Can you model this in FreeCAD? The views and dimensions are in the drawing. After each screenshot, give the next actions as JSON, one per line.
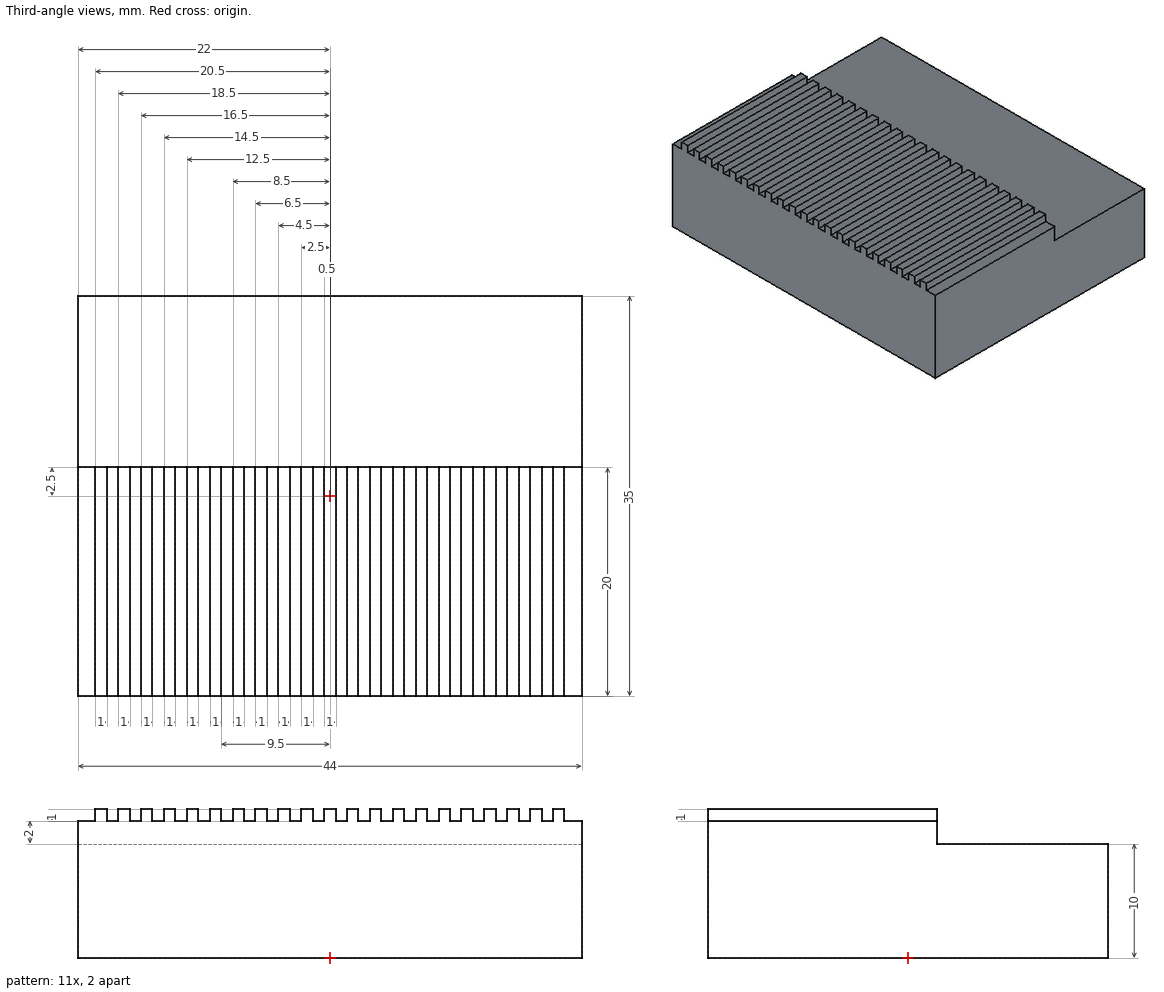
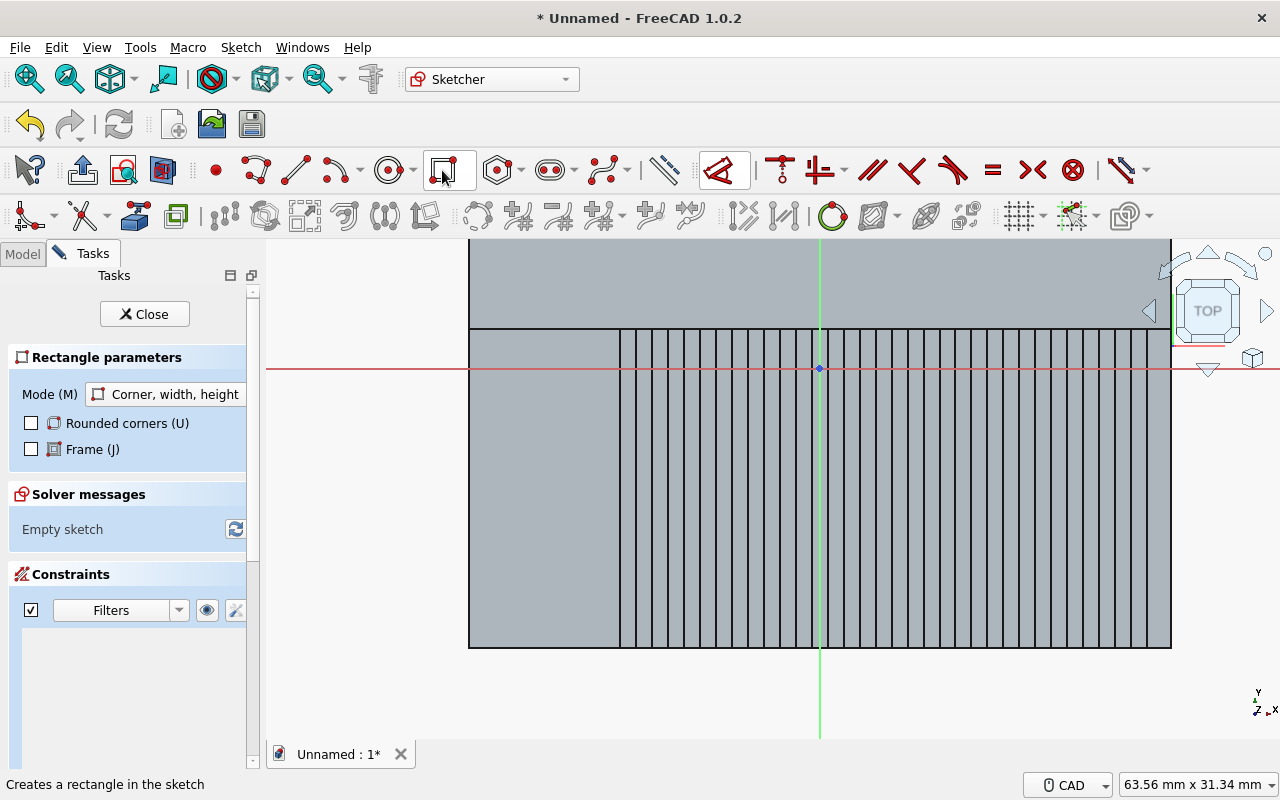
{"action": "left_click", "coordinate": [589, 329]}
{"action": "mouse_move", "coordinate": [604, 648]}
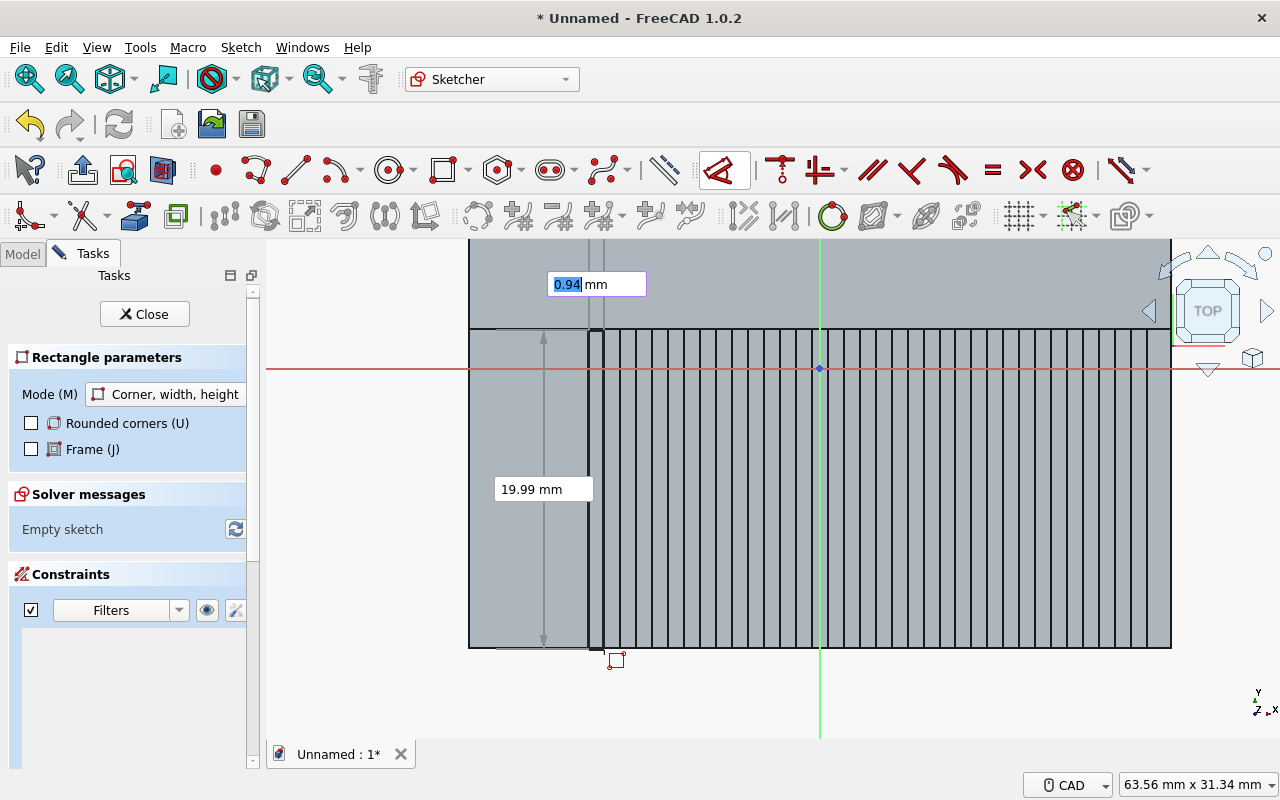
{"action": "type", "text": "1"}
{"action": "key", "text": "Tab"}
{"action": "type", "text": "20"}
{"action": "key", "text": "Return"}
{"action": "key", "text": "Escape"}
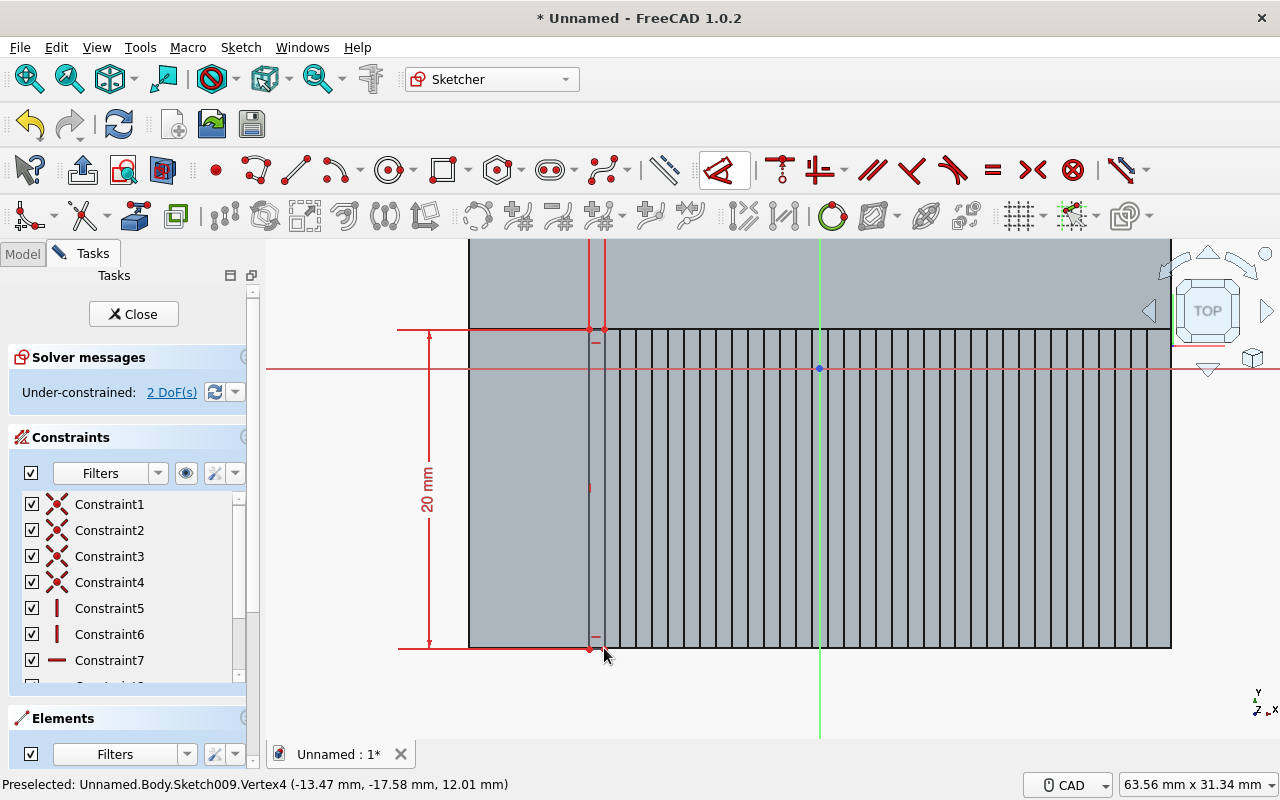
{"action": "left_click", "coordinate": [589, 330]}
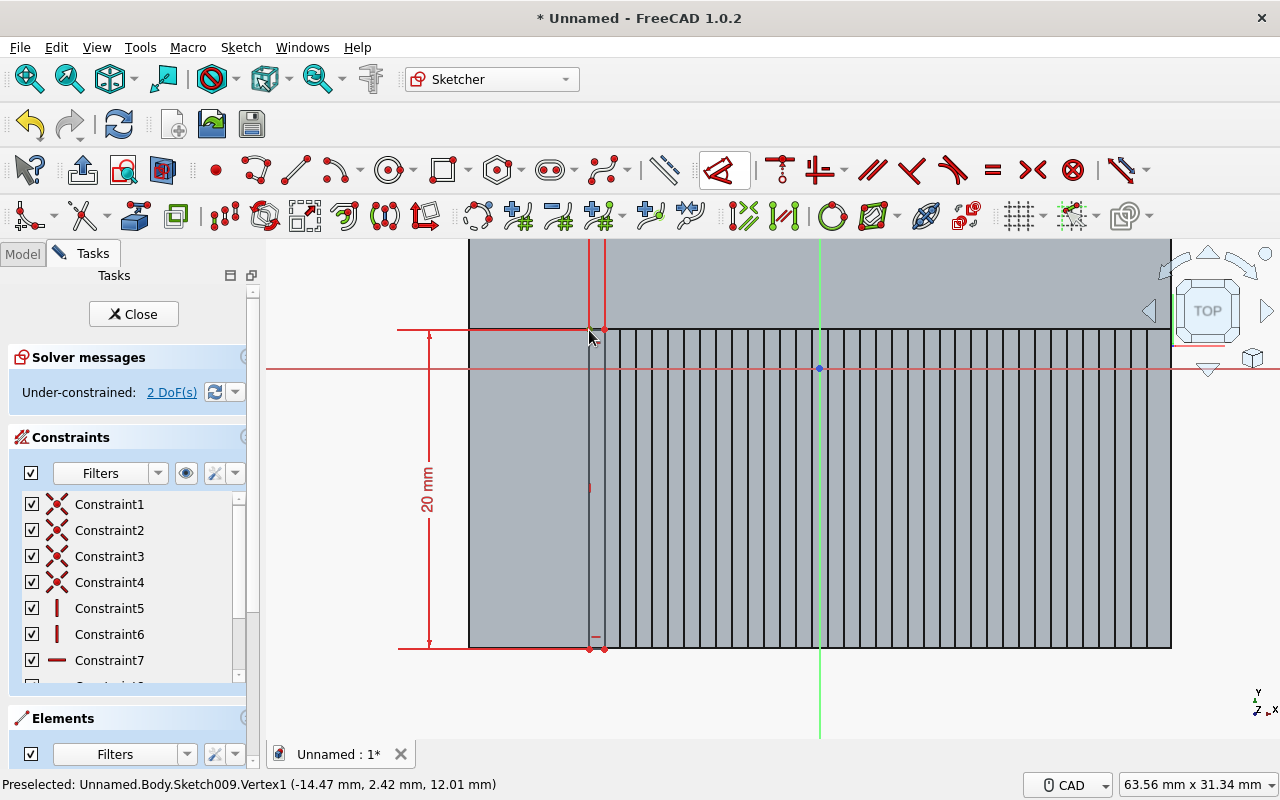
{"action": "left_click", "coordinate": [744, 170]}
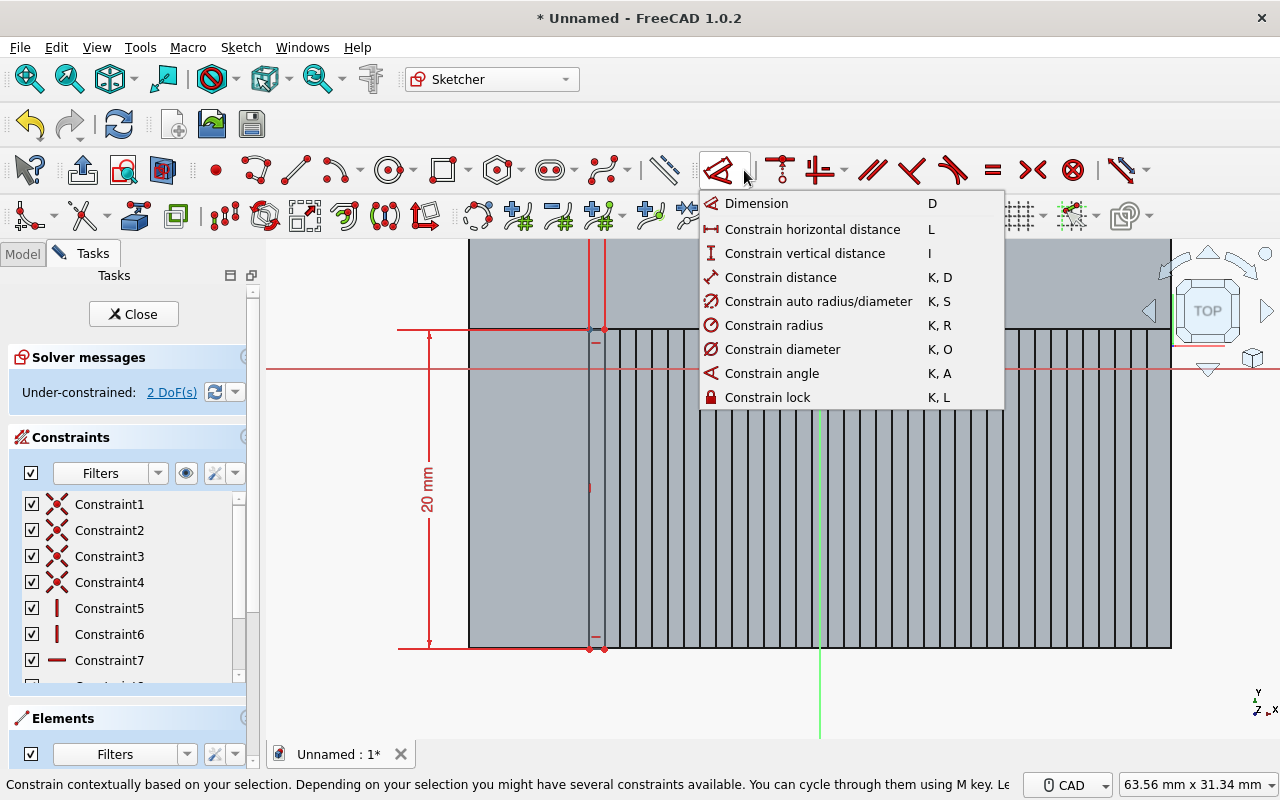
{"action": "left_click", "coordinate": [852, 253]}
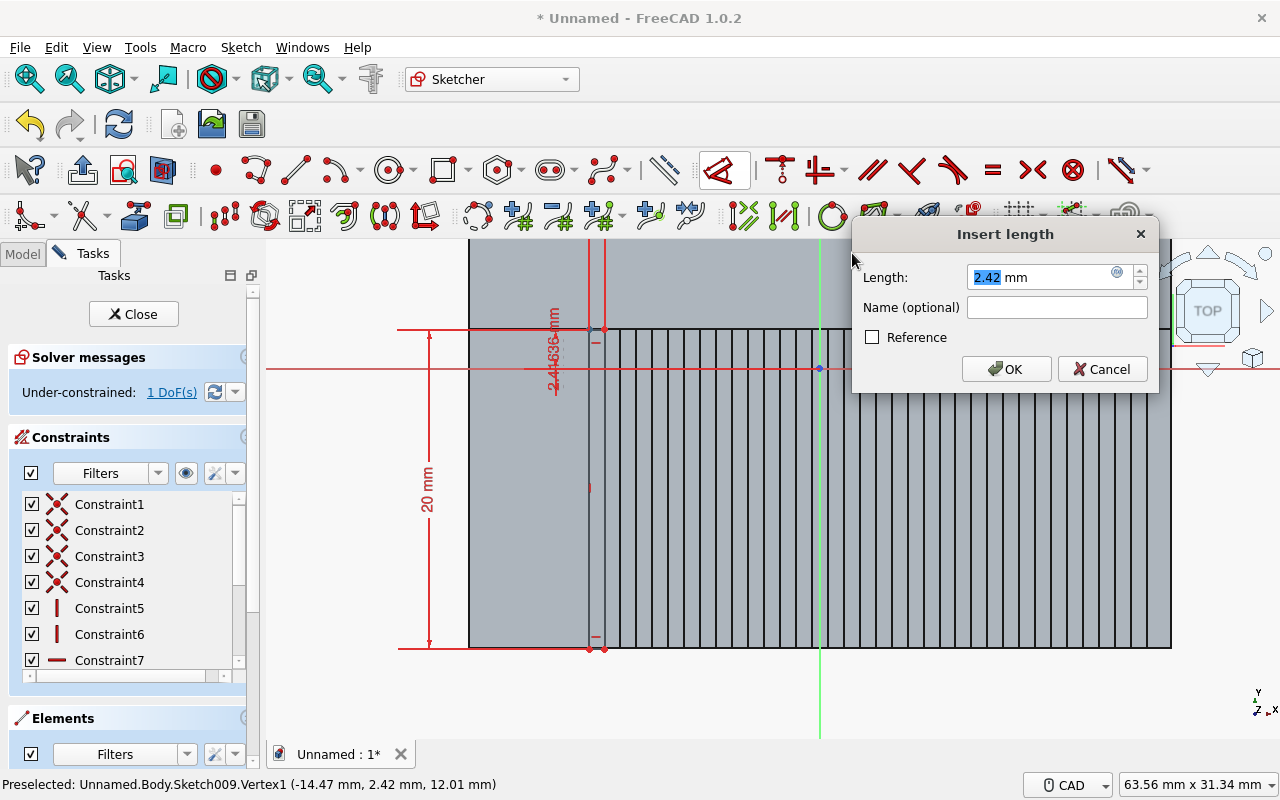
{"action": "type", "text": "2.5"}
{"action": "key", "text": "Return"}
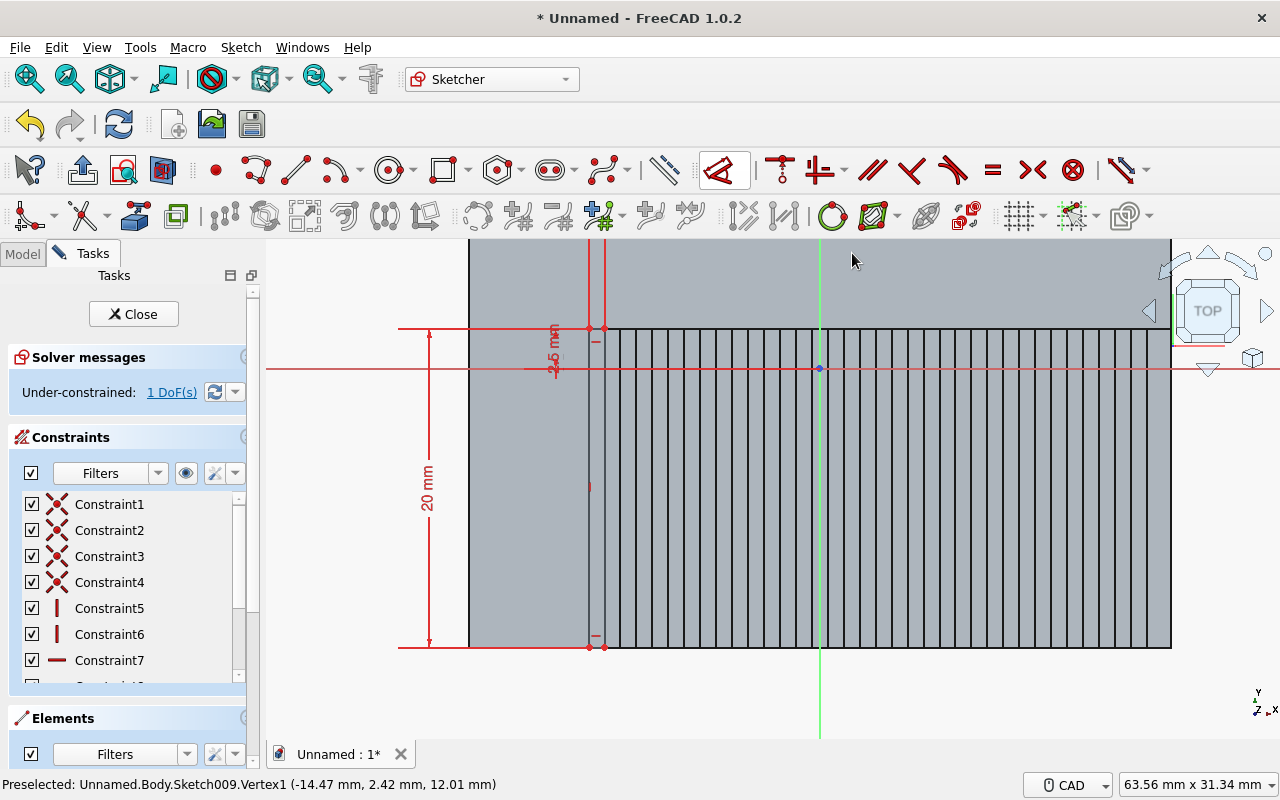
{"action": "left_click", "coordinate": [589, 329]}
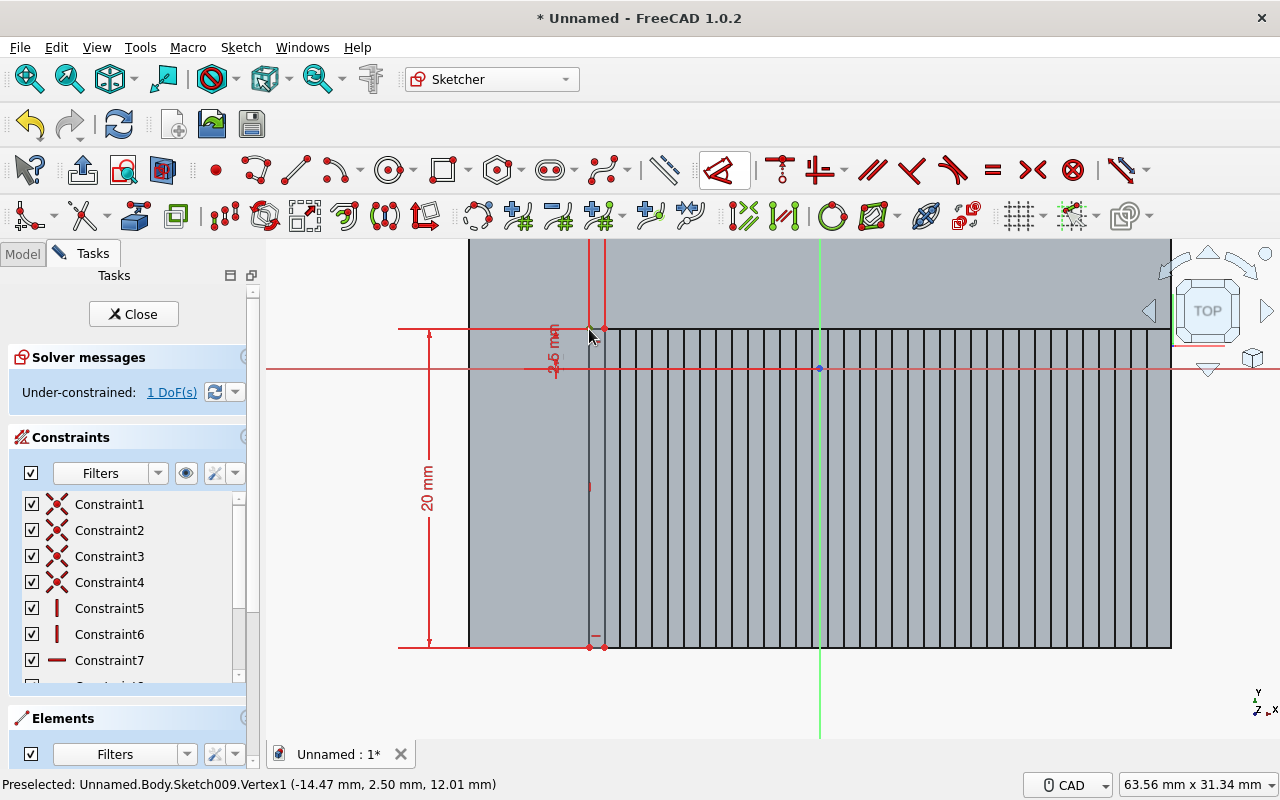
{"action": "left_click", "coordinate": [744, 170]}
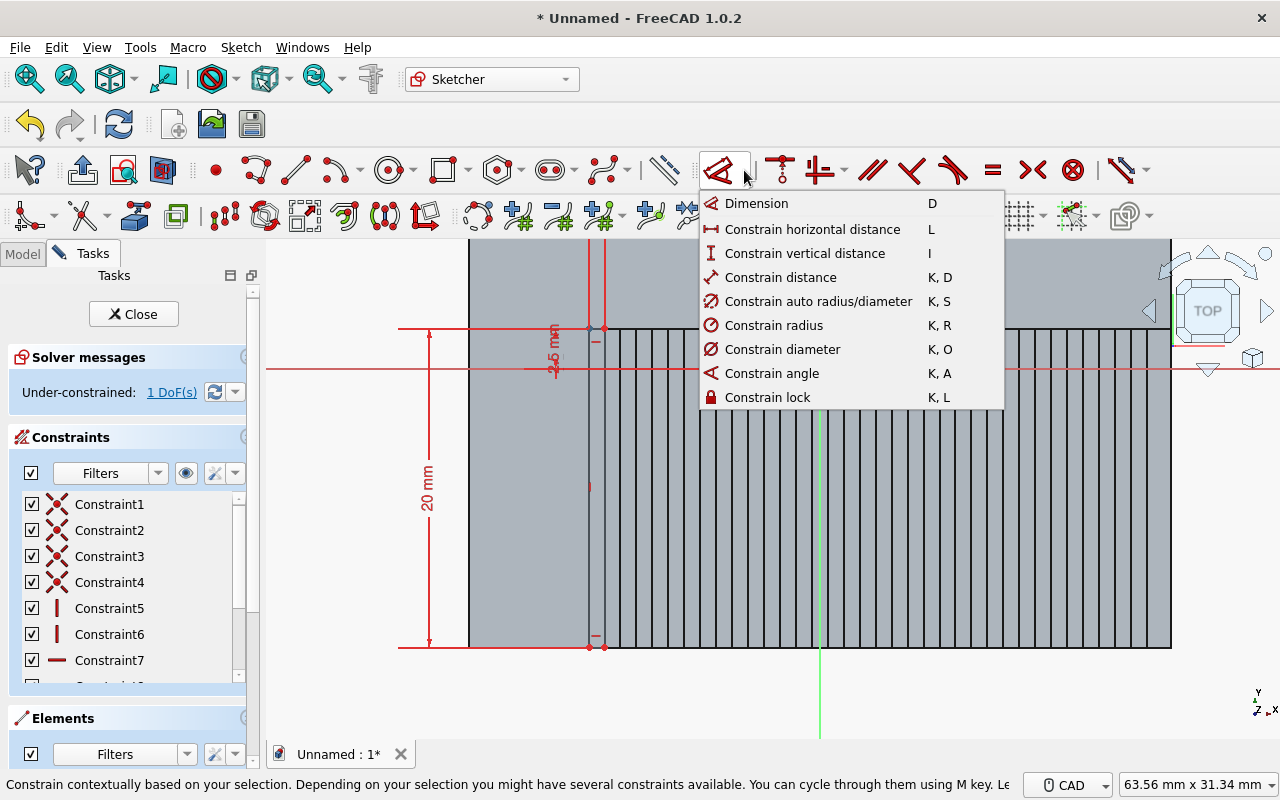
{"action": "left_click", "coordinate": [852, 229]}